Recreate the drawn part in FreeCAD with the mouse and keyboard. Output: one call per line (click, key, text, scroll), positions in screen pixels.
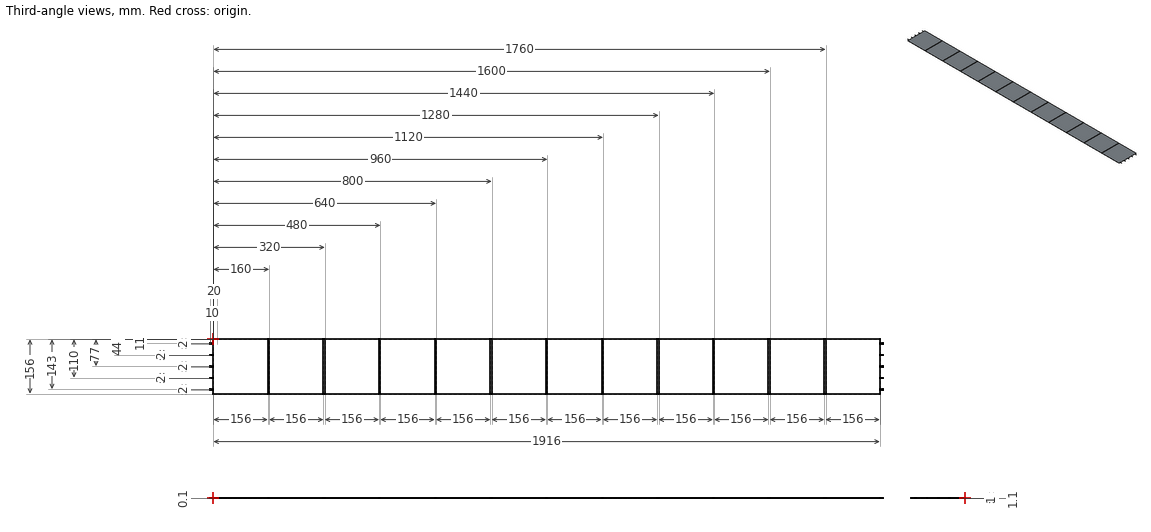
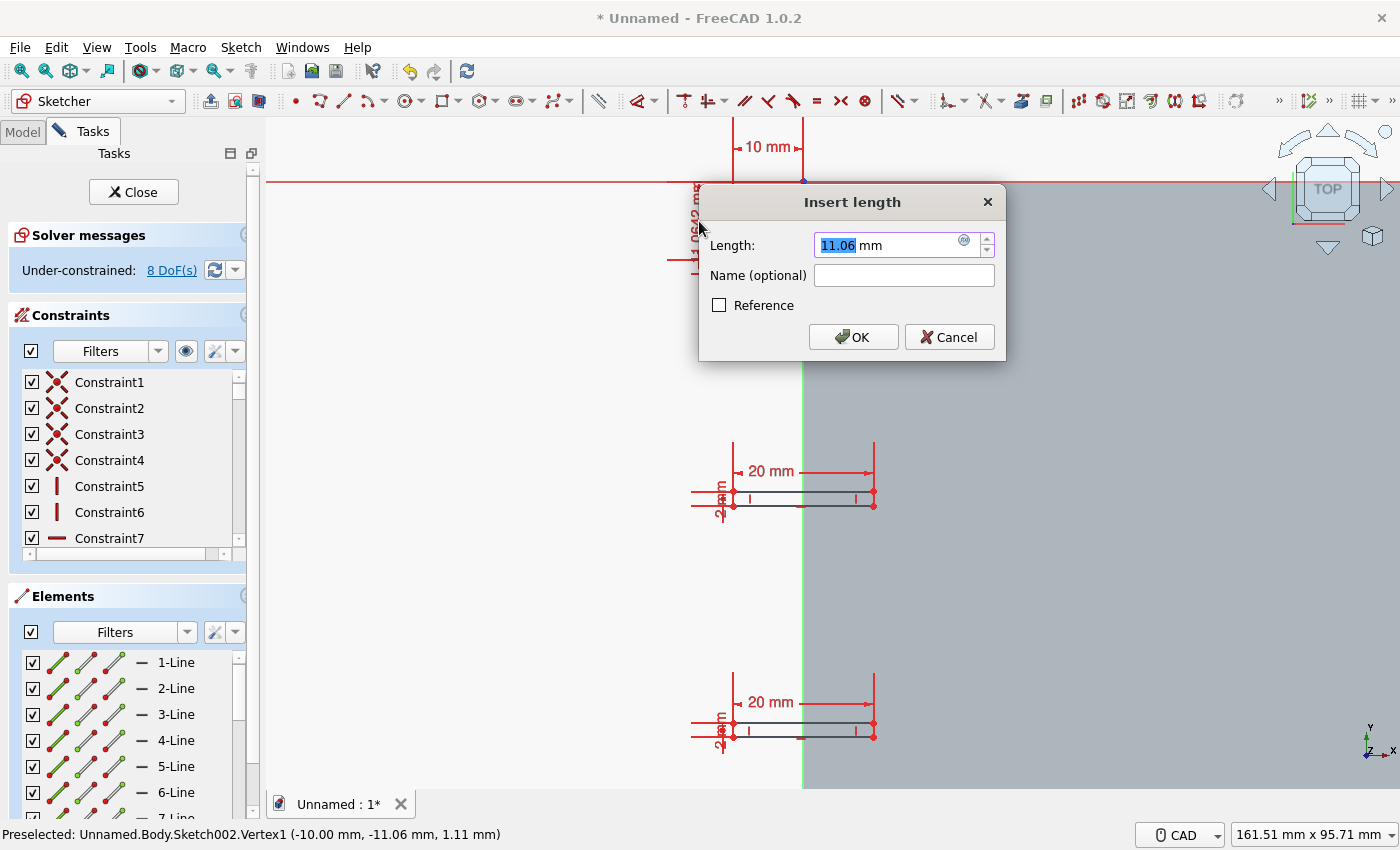
text(11)
key(Return)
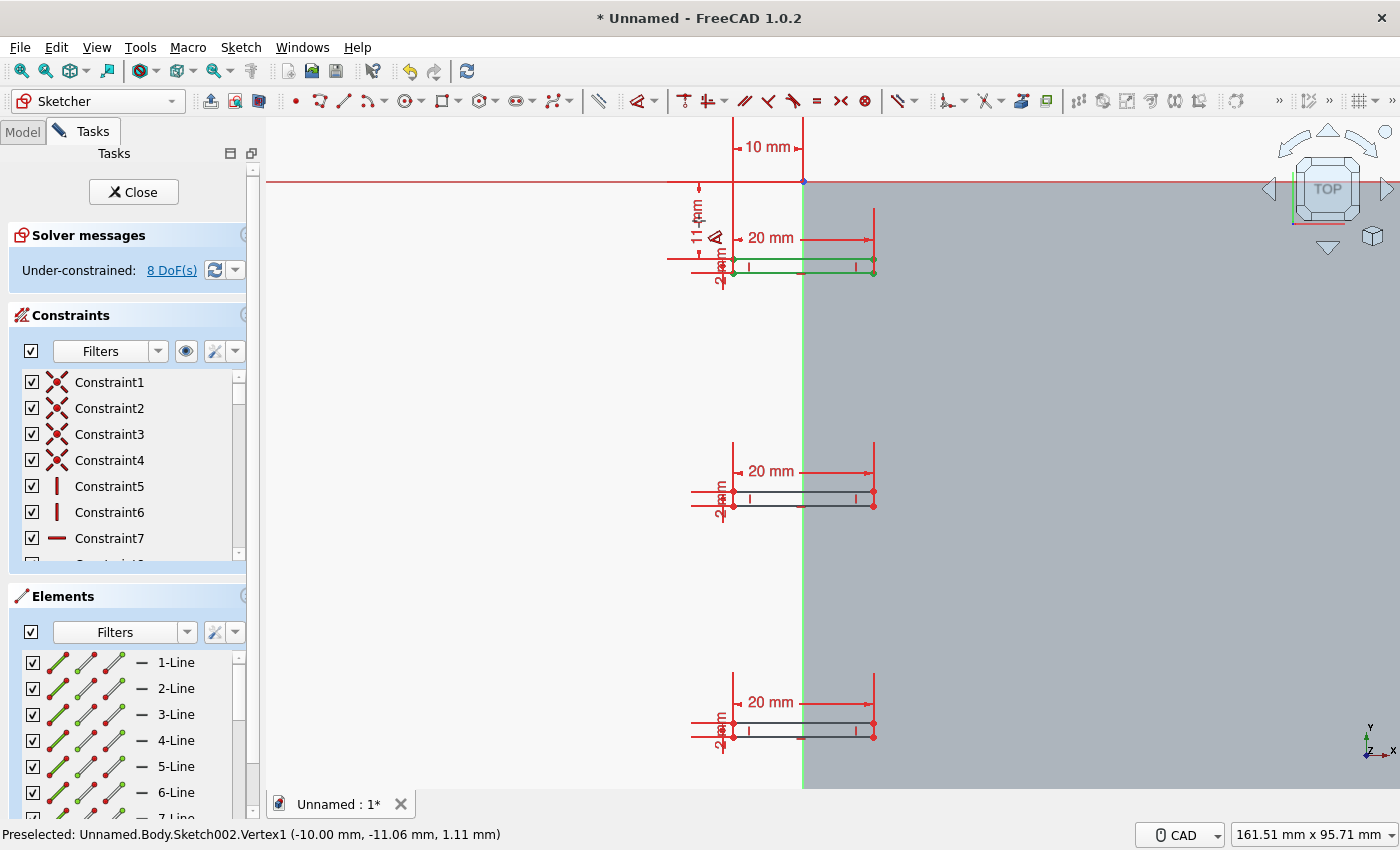
click(733, 492)
click(768, 526)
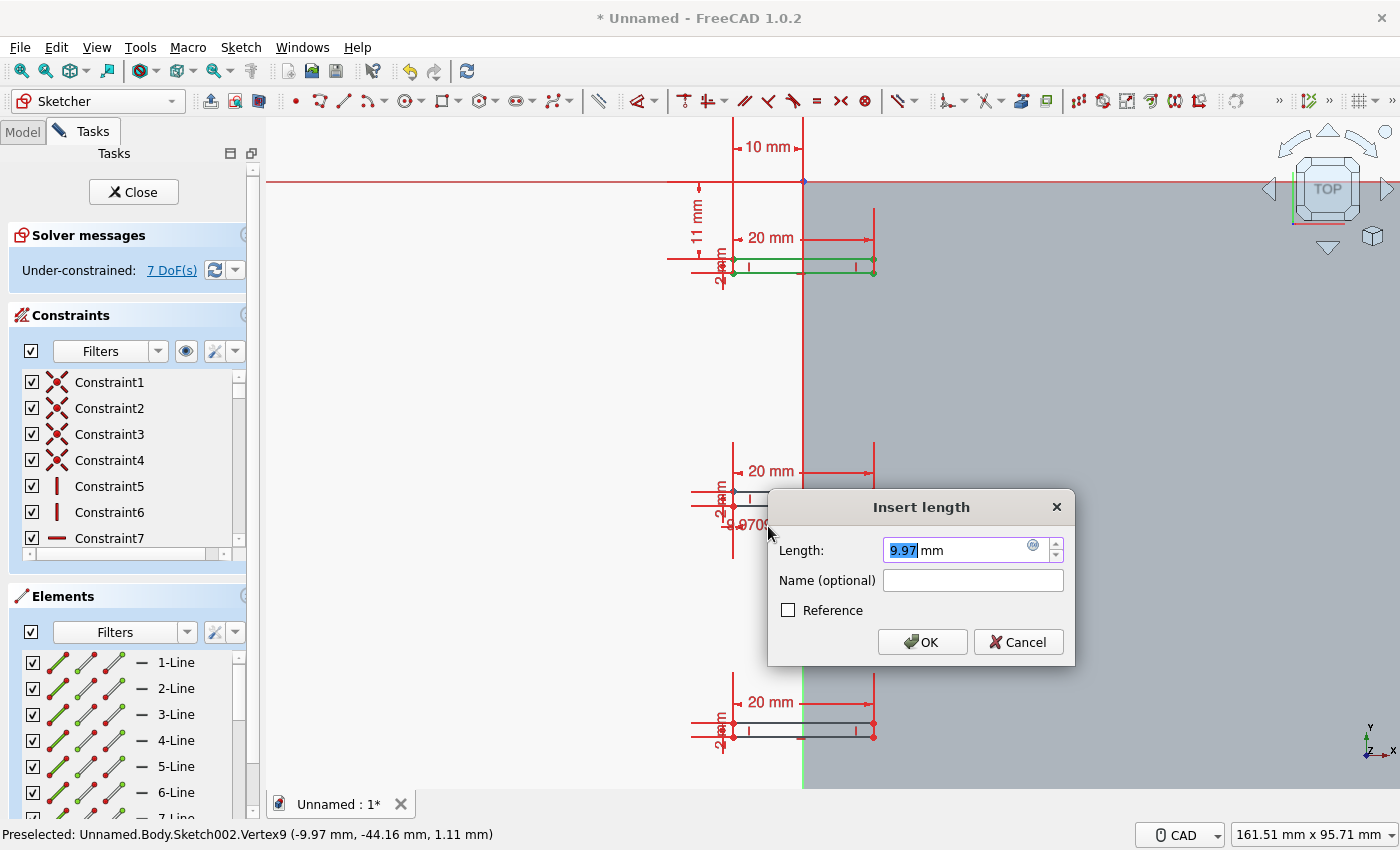
text(10)
key(Return)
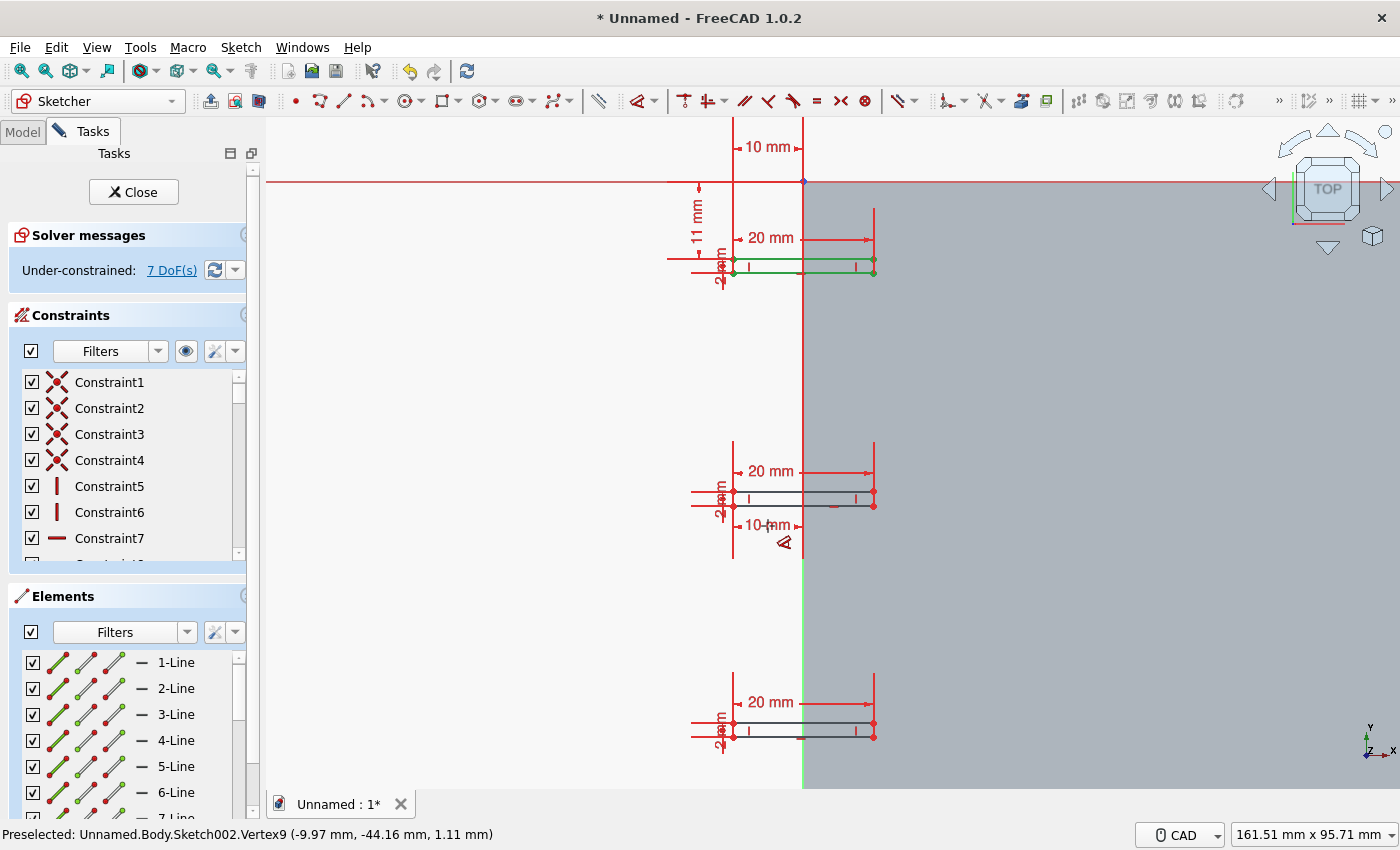
click(733, 492)
click(699, 337)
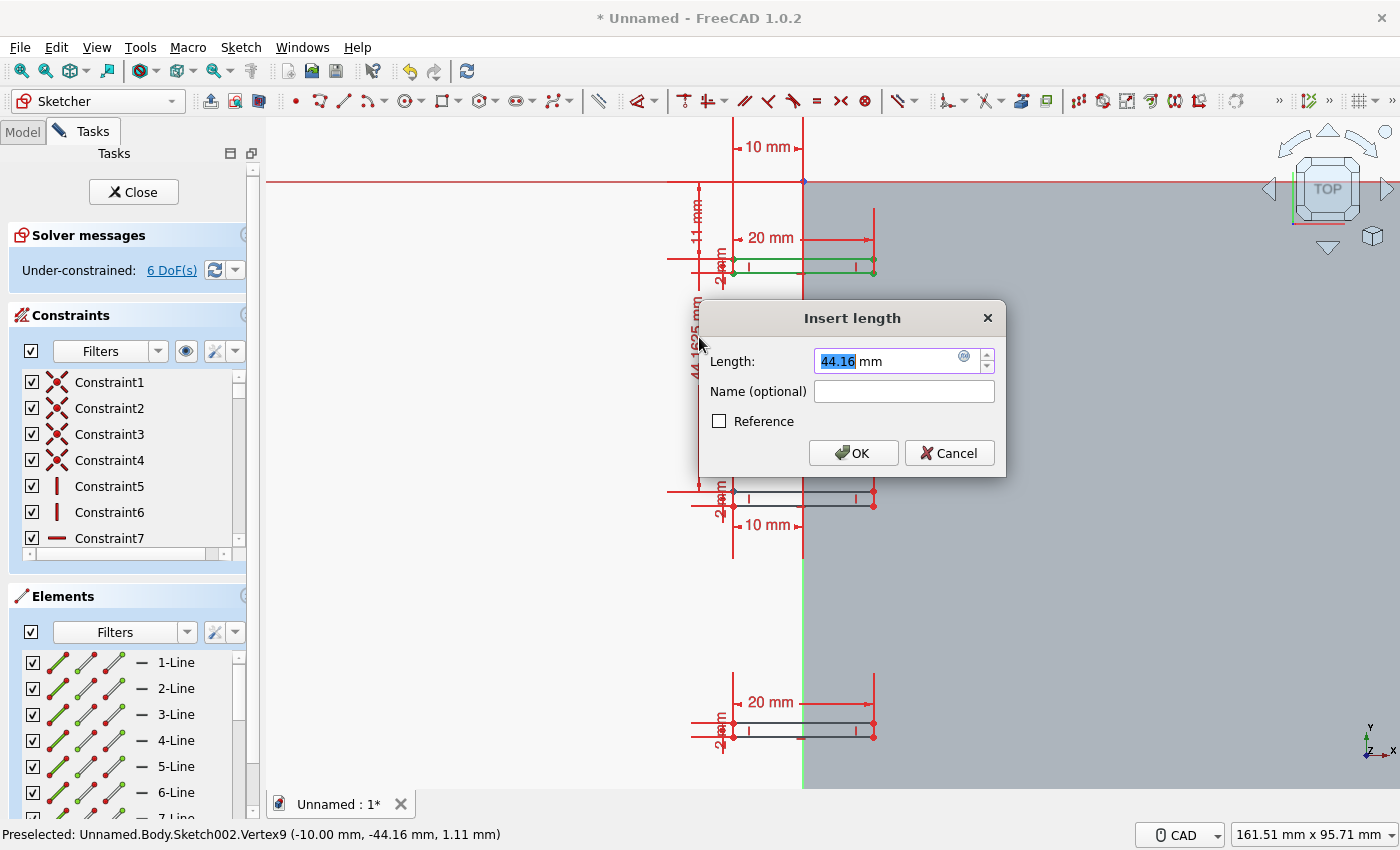
text(44)
key(Return)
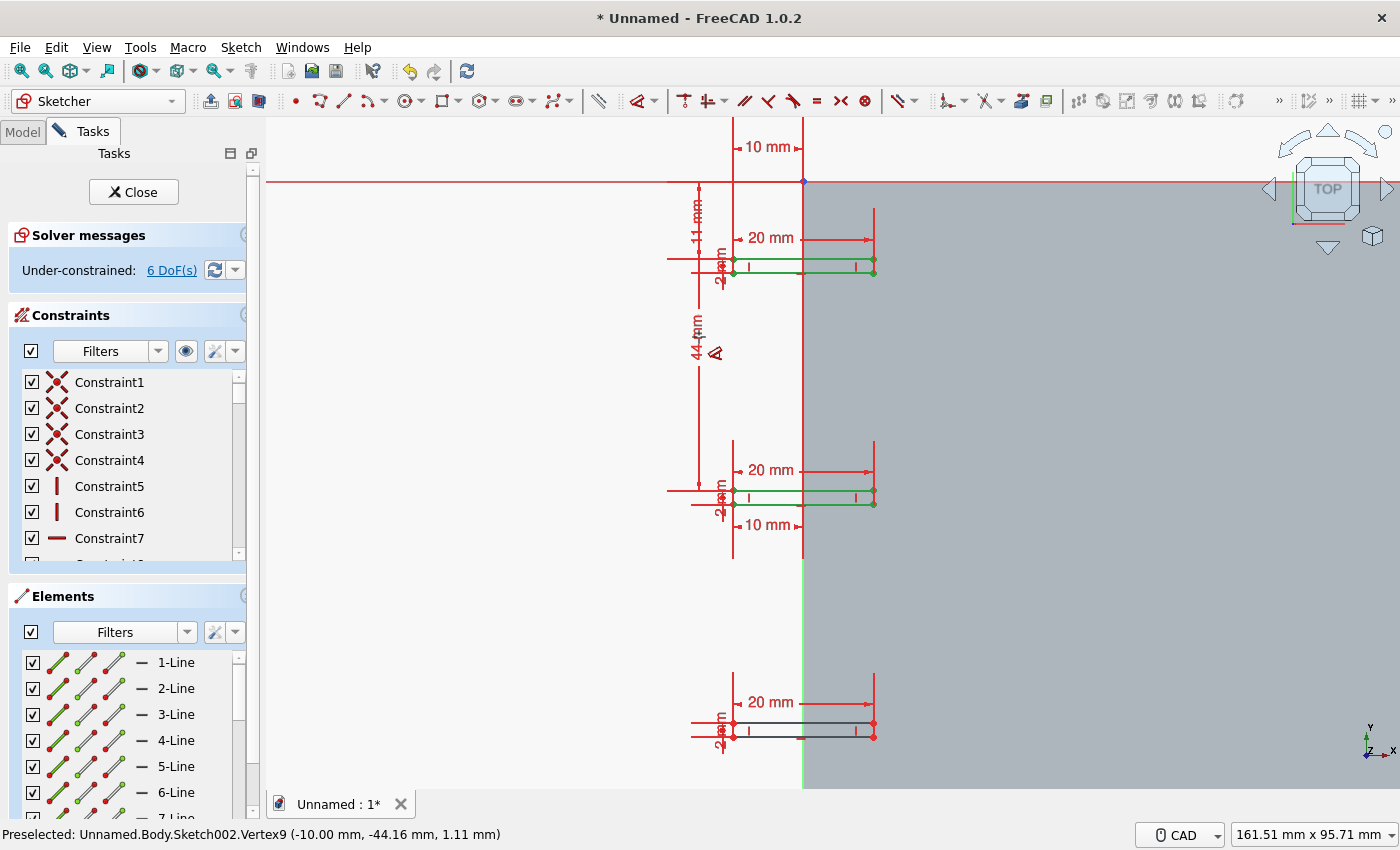
click(733, 723)
click(768, 757)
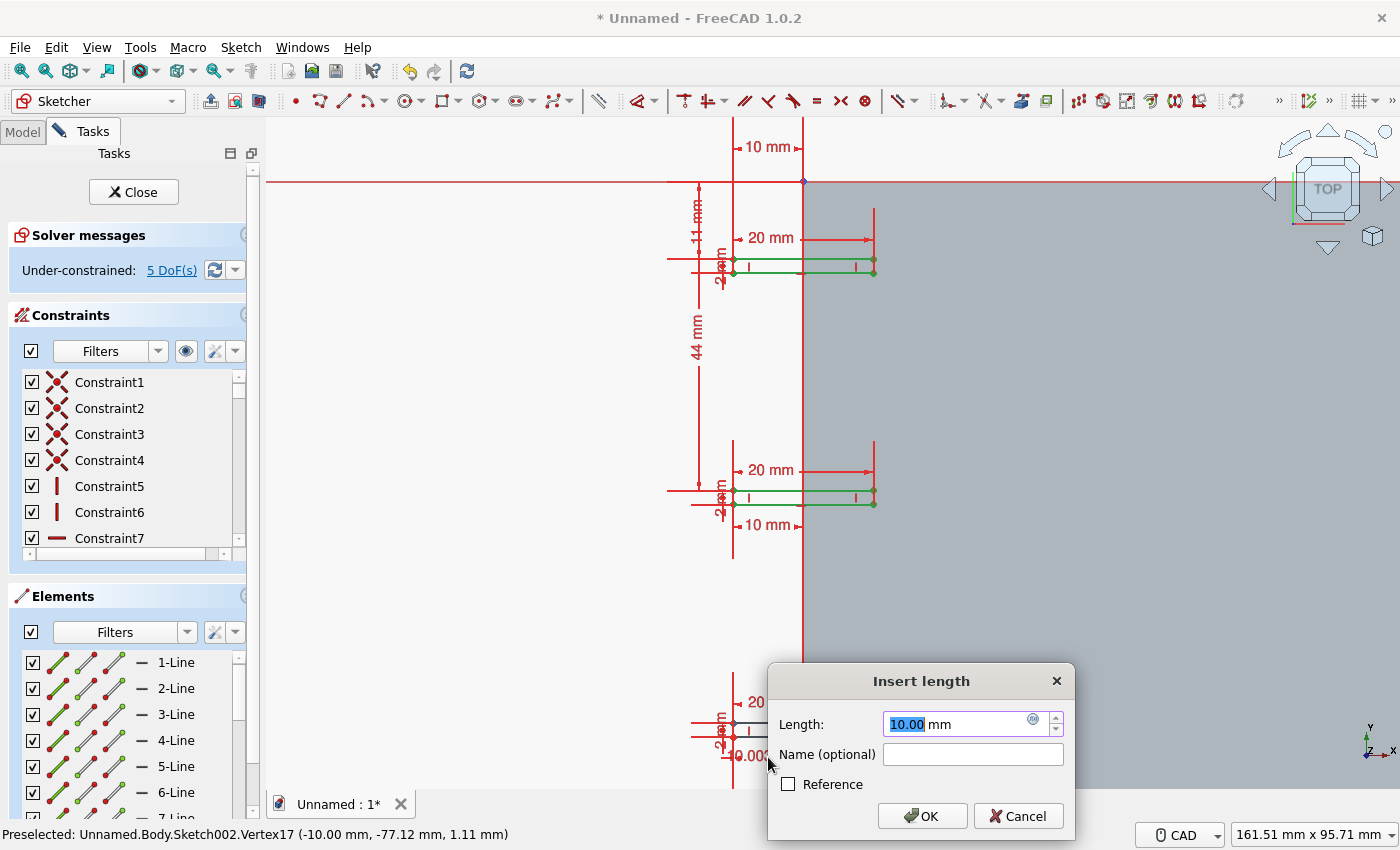
text(10)
key(Return)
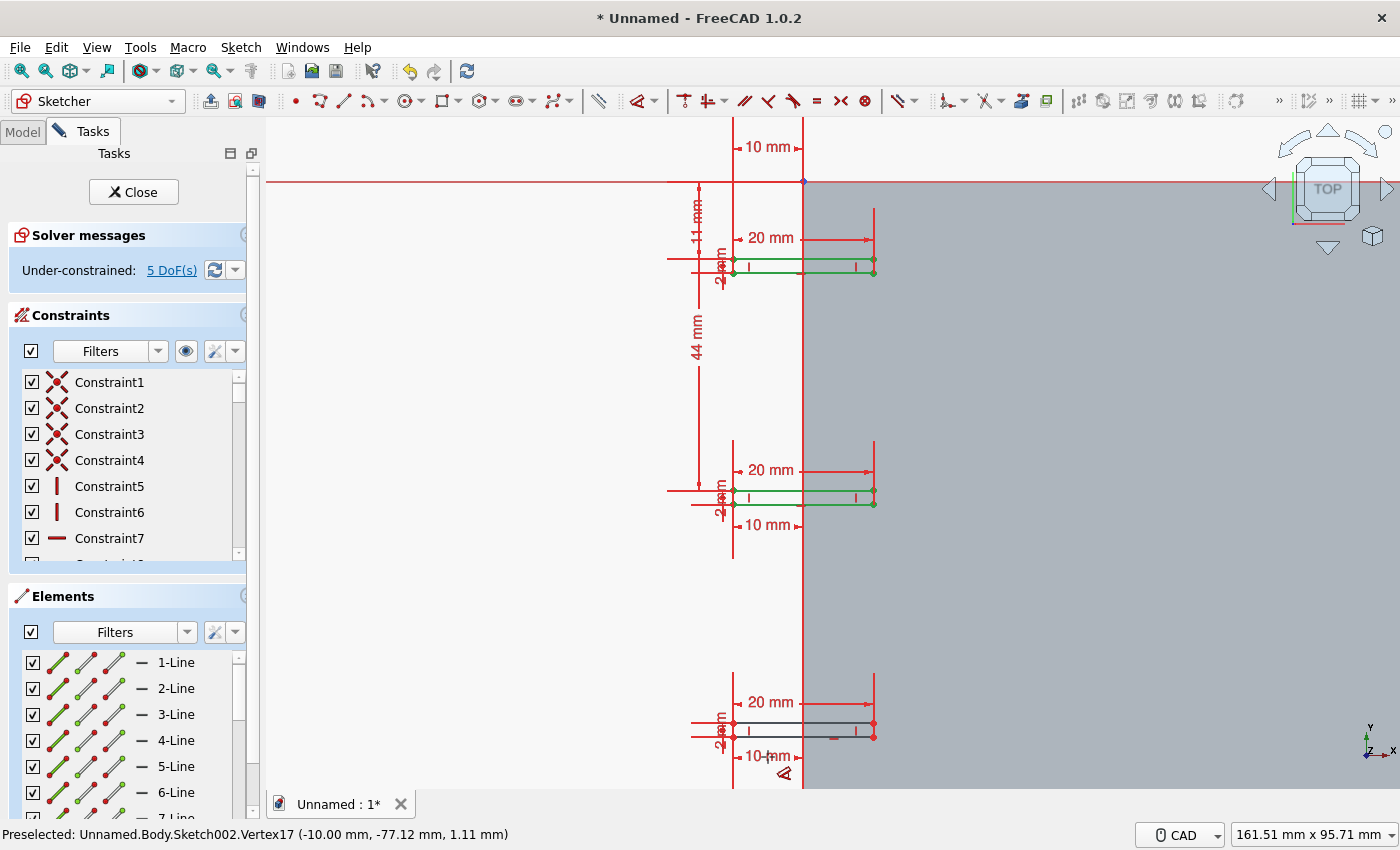
click(733, 723)
click(699, 453)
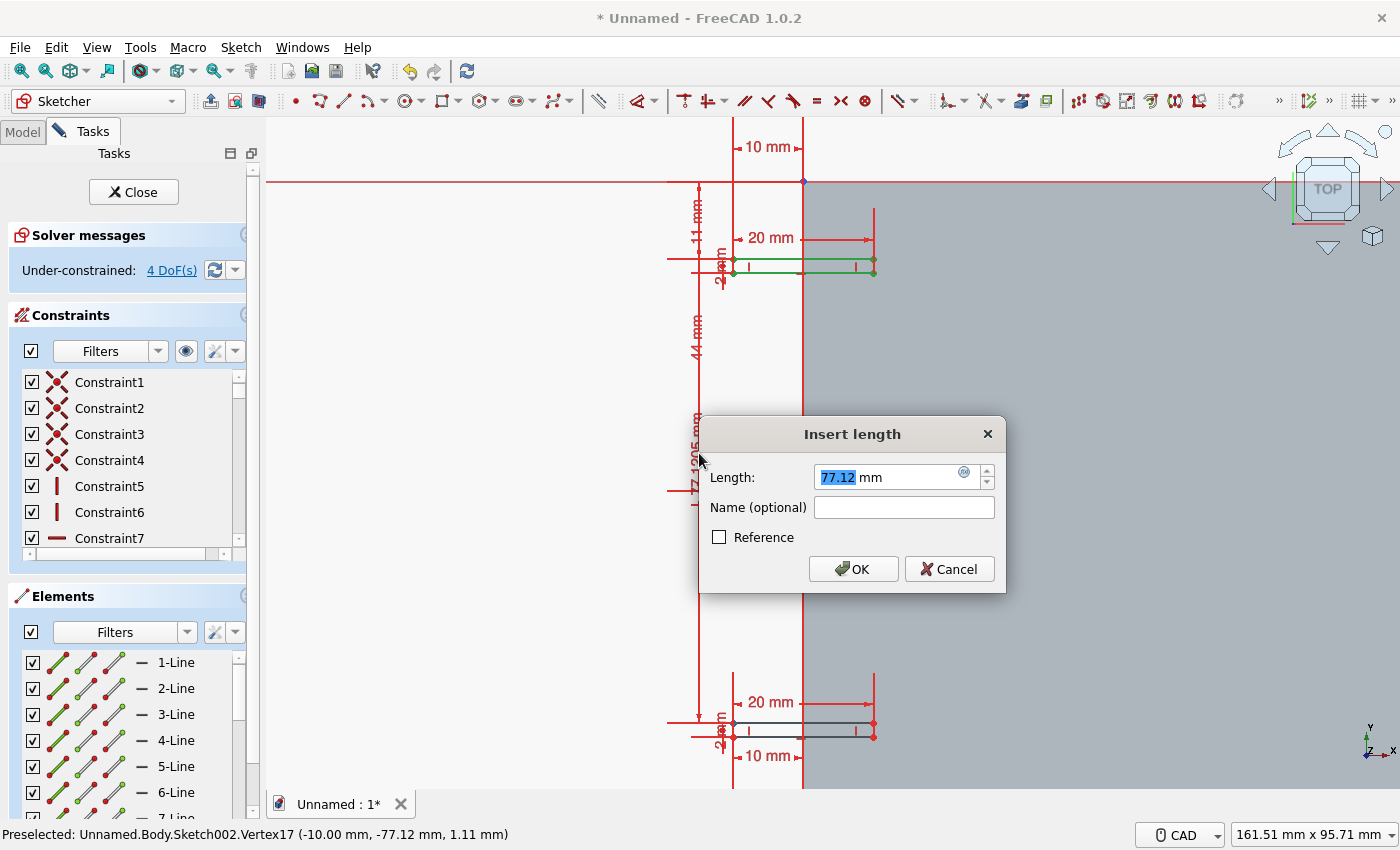
text(77)
key(Return)